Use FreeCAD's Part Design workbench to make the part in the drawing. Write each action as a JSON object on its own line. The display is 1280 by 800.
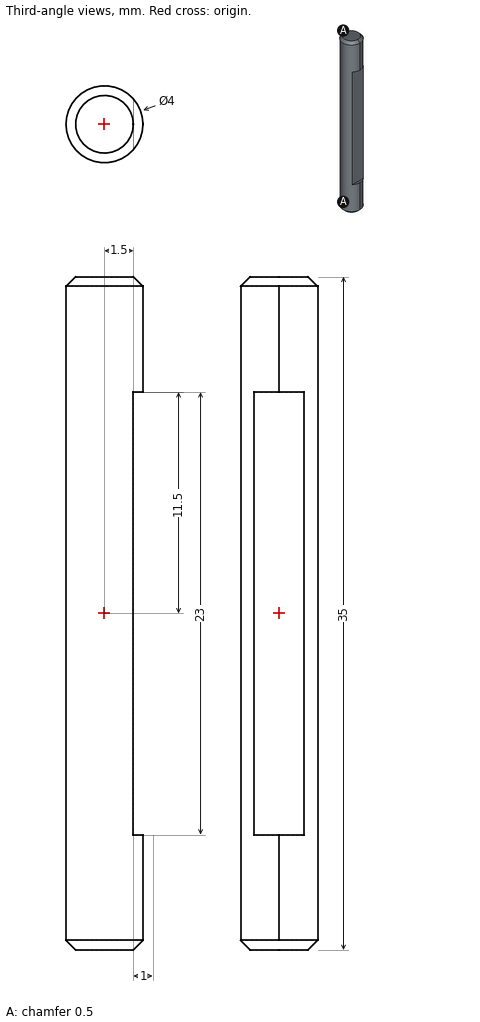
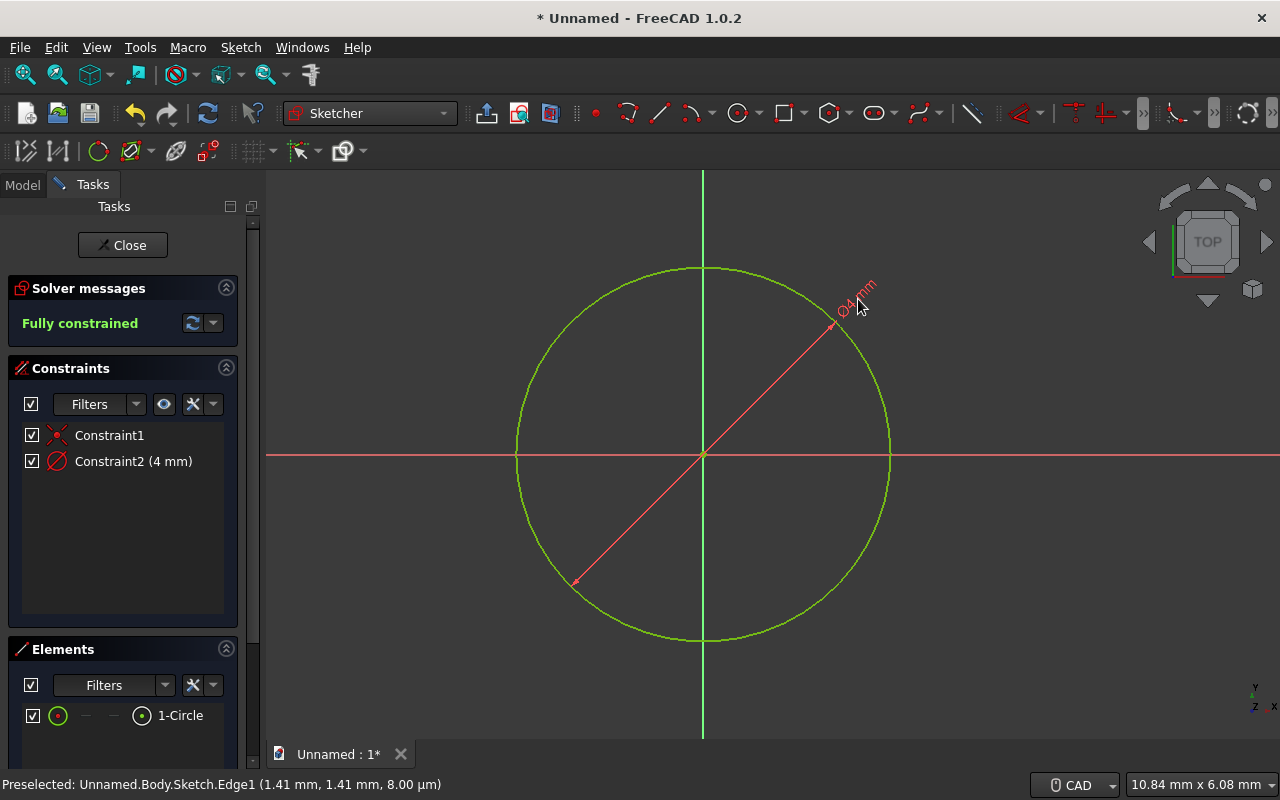
{"action": "left_click", "coordinate": [123, 245]}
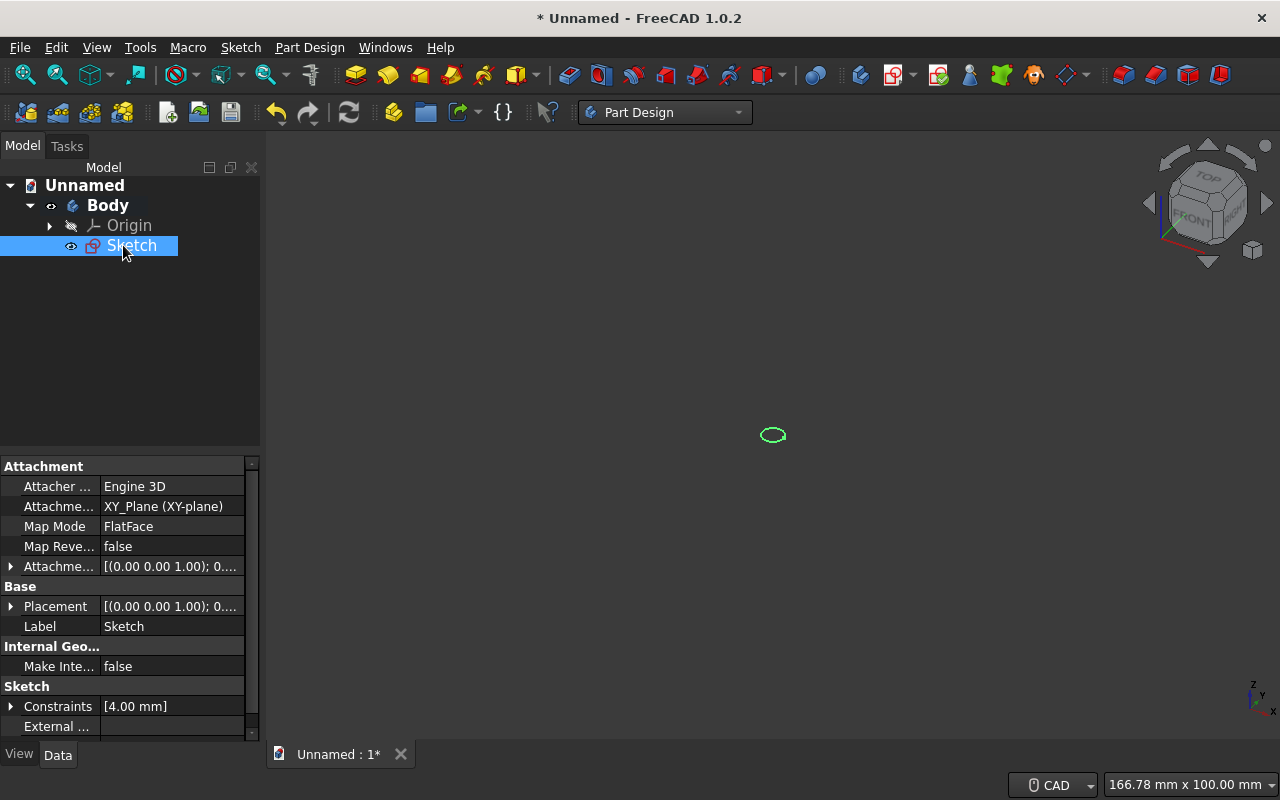
{"action": "left_click", "coordinate": [356, 76]}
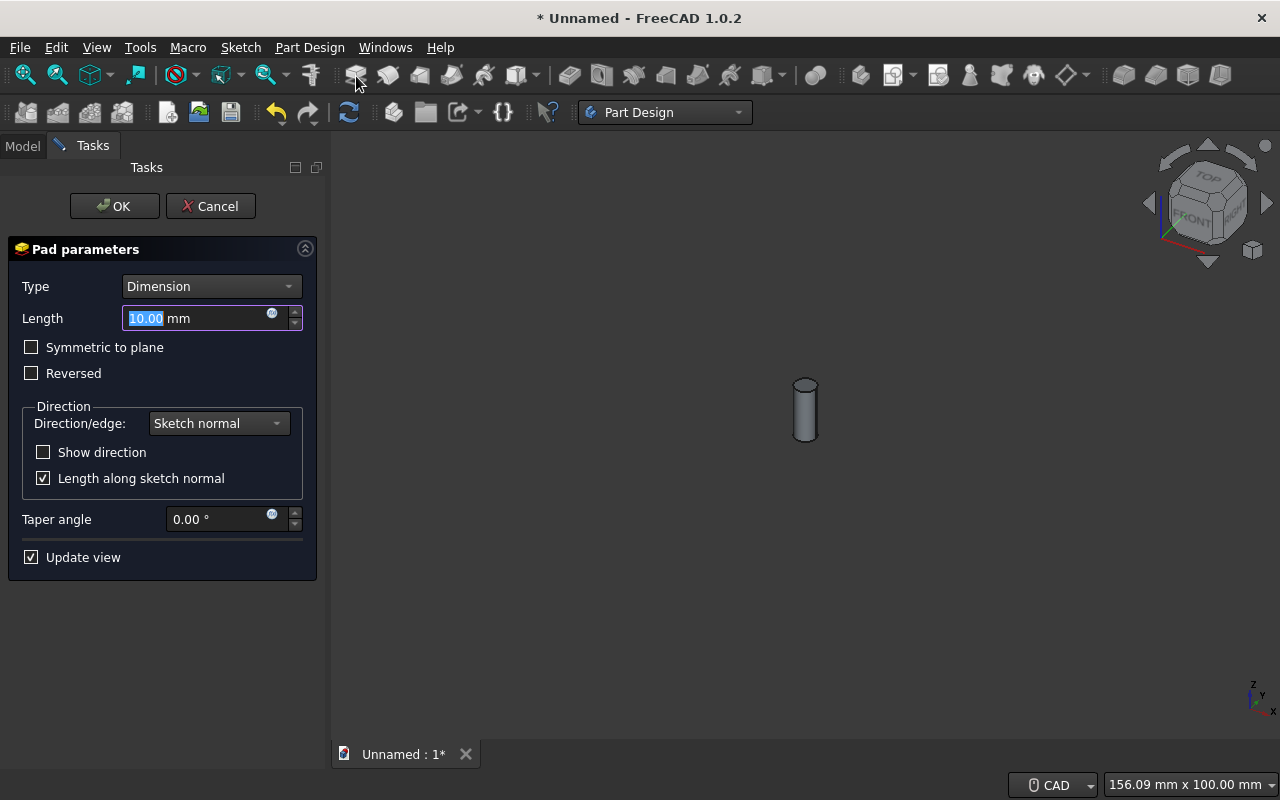
{"action": "type", "text": "35"}
{"action": "key", "text": "Tab"}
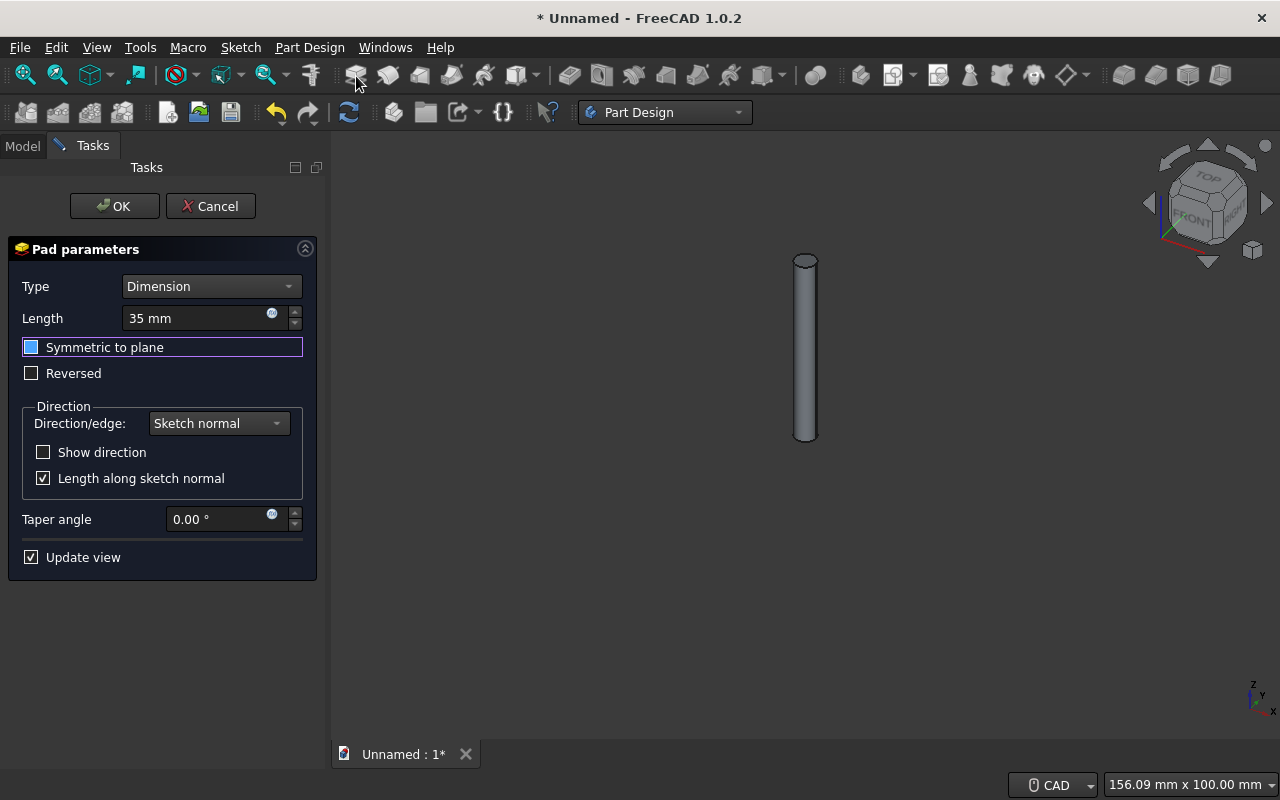
{"action": "left_click", "coordinate": [30, 347]}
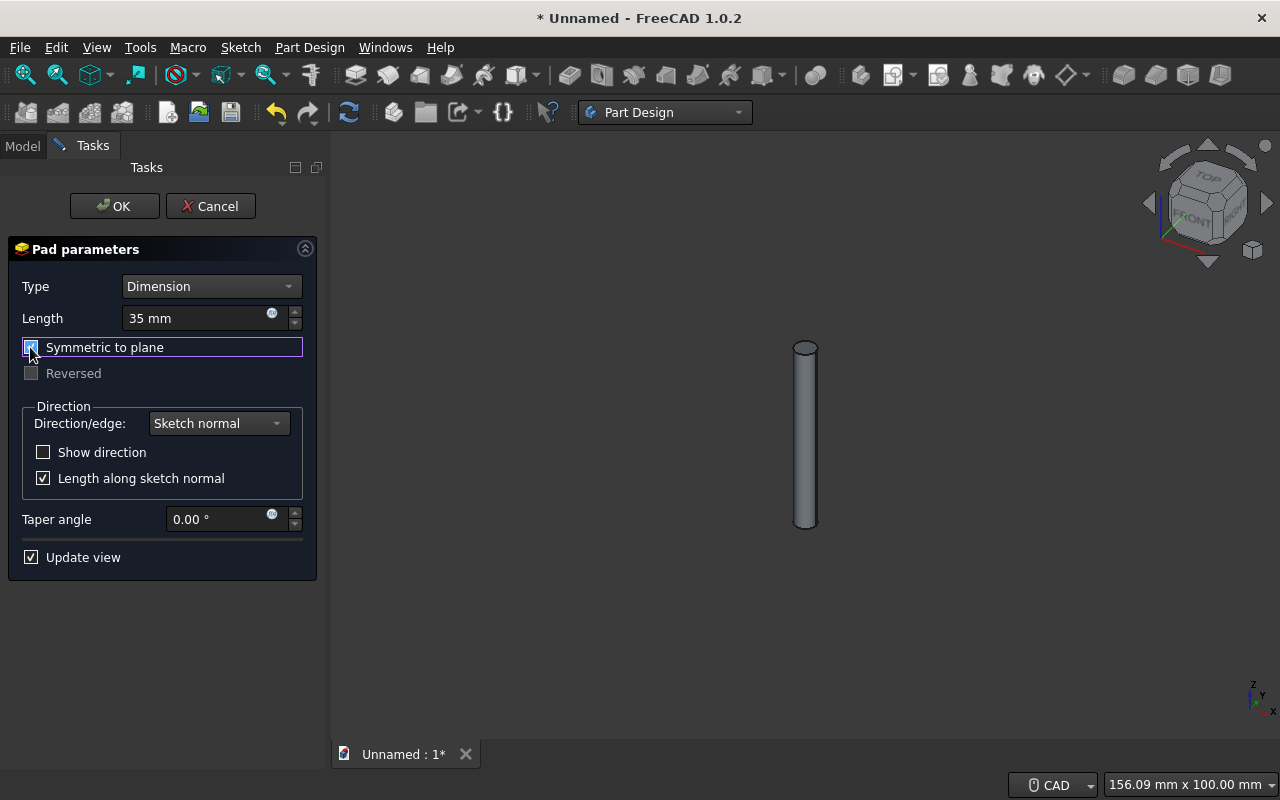
{"action": "left_click", "coordinate": [115, 206]}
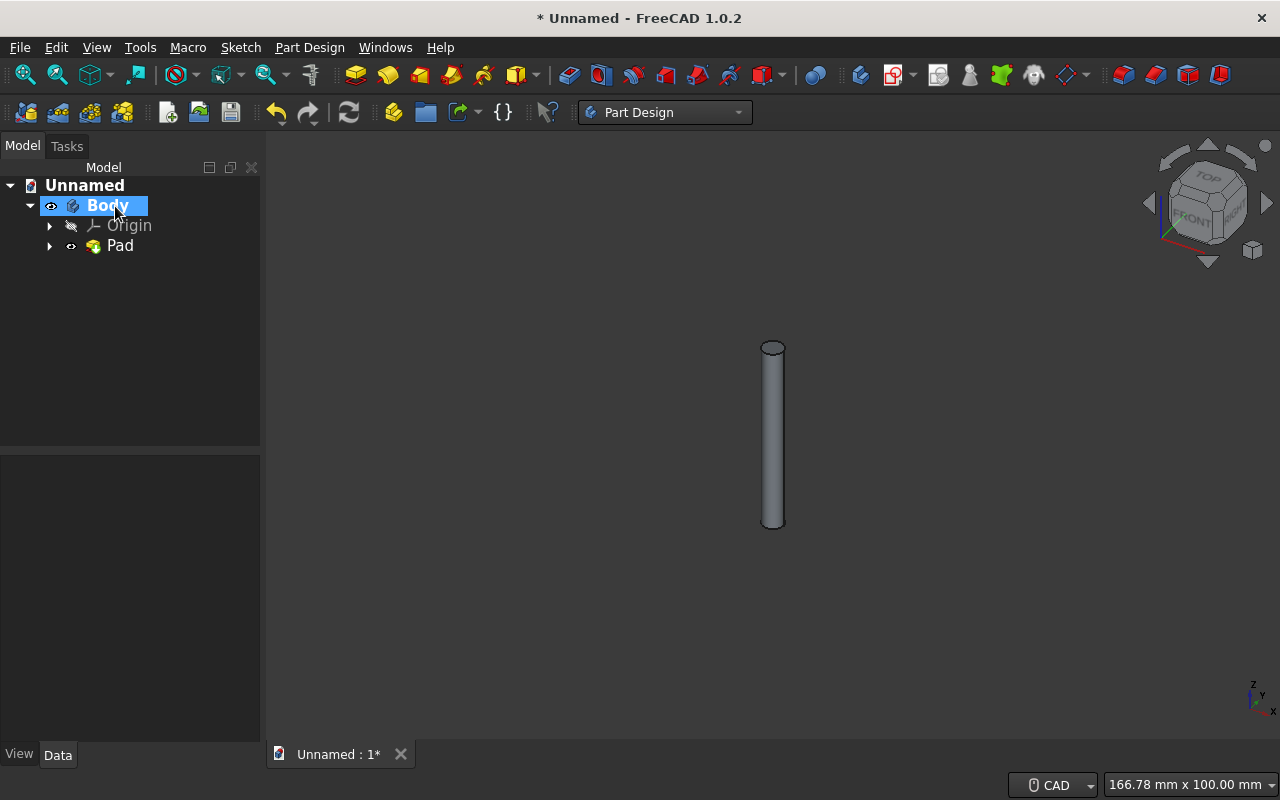
{"action": "key", "text": "v f"}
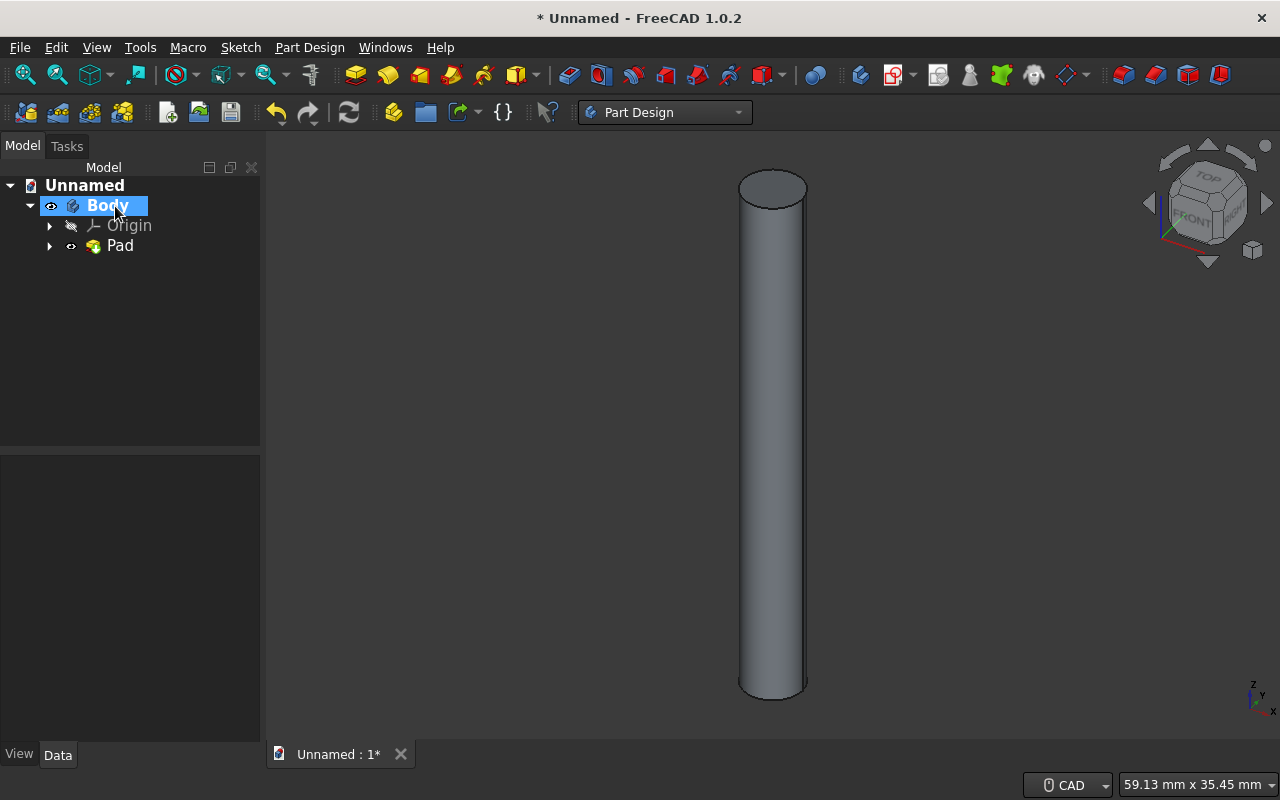
{"action": "left_click", "coordinate": [743, 178]}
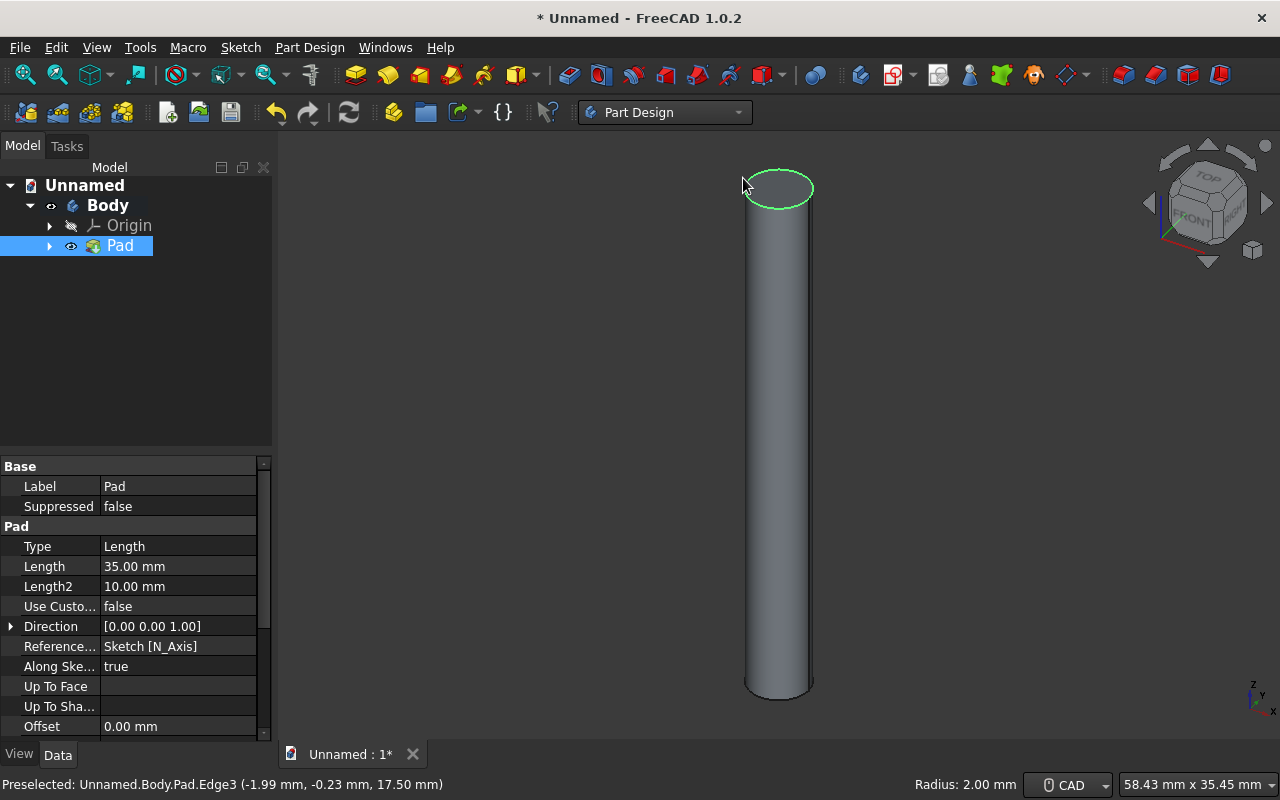
{"action": "key", "text": "0"}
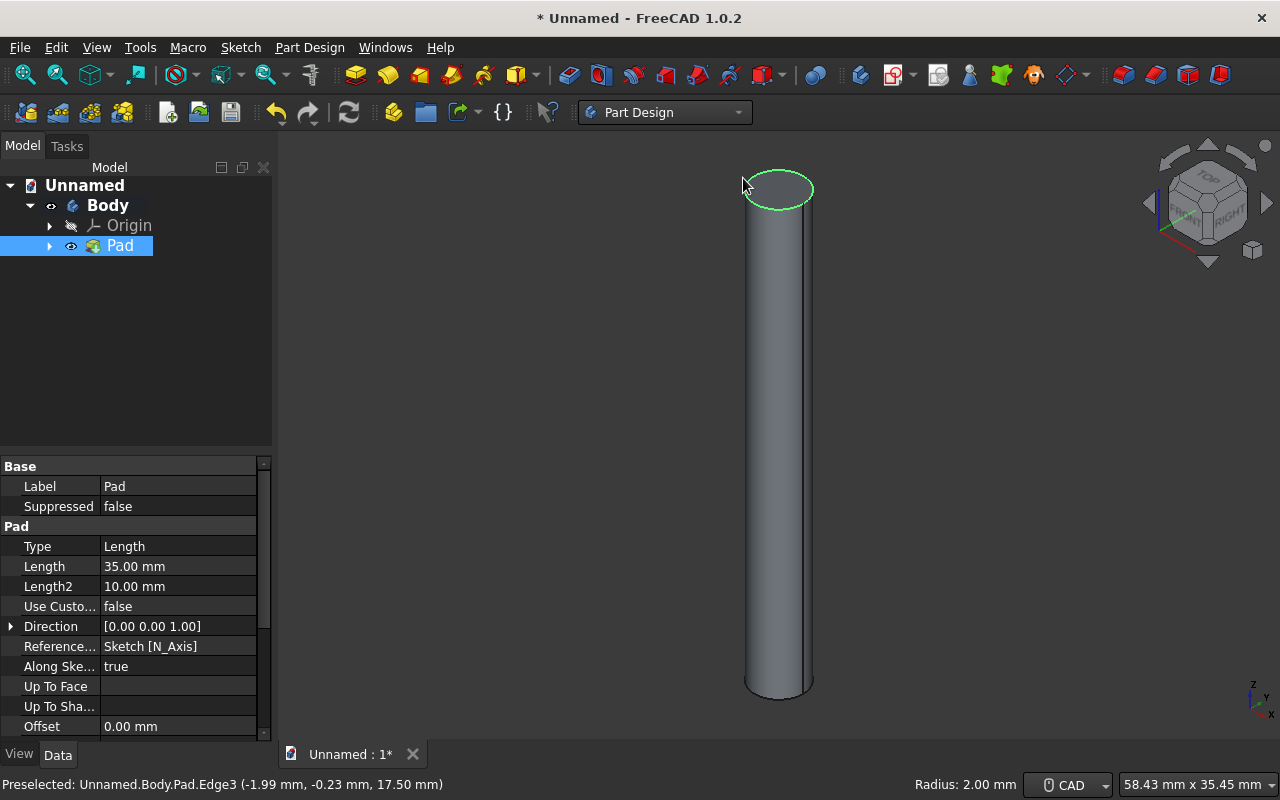
{"action": "left_click", "coordinate": [763, 697], "text": "ctrl"}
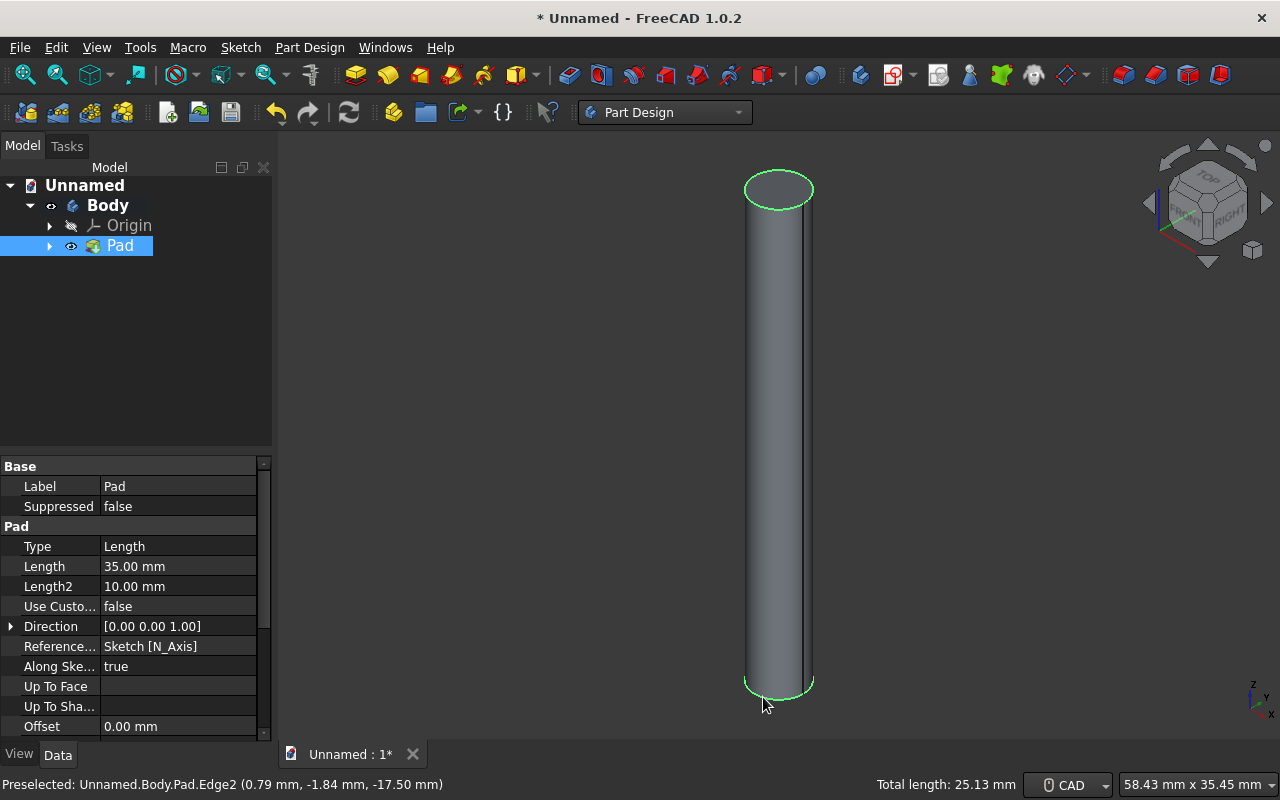
{"action": "left_click", "coordinate": [1156, 76]}